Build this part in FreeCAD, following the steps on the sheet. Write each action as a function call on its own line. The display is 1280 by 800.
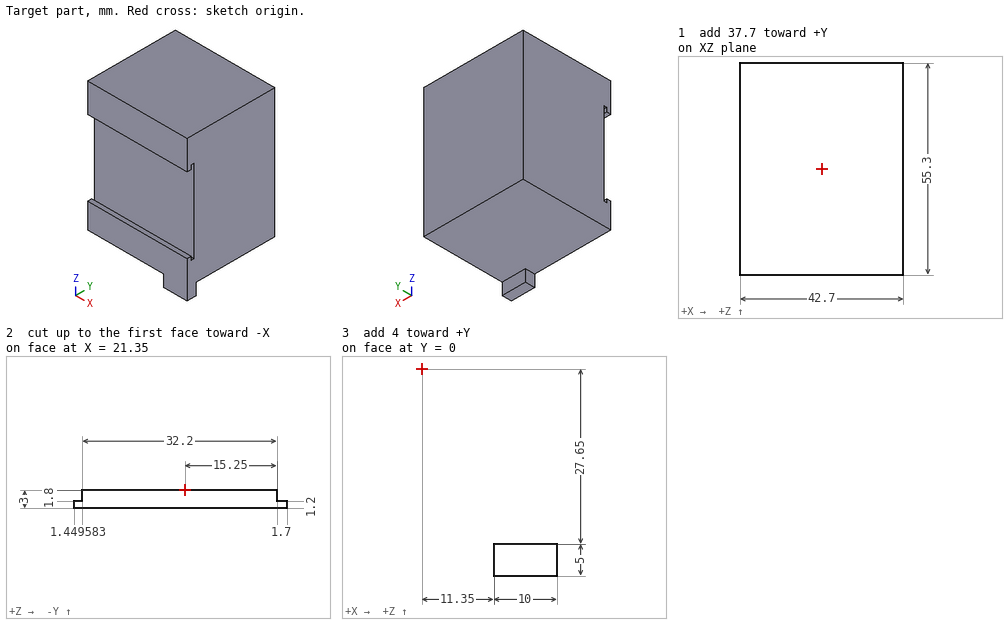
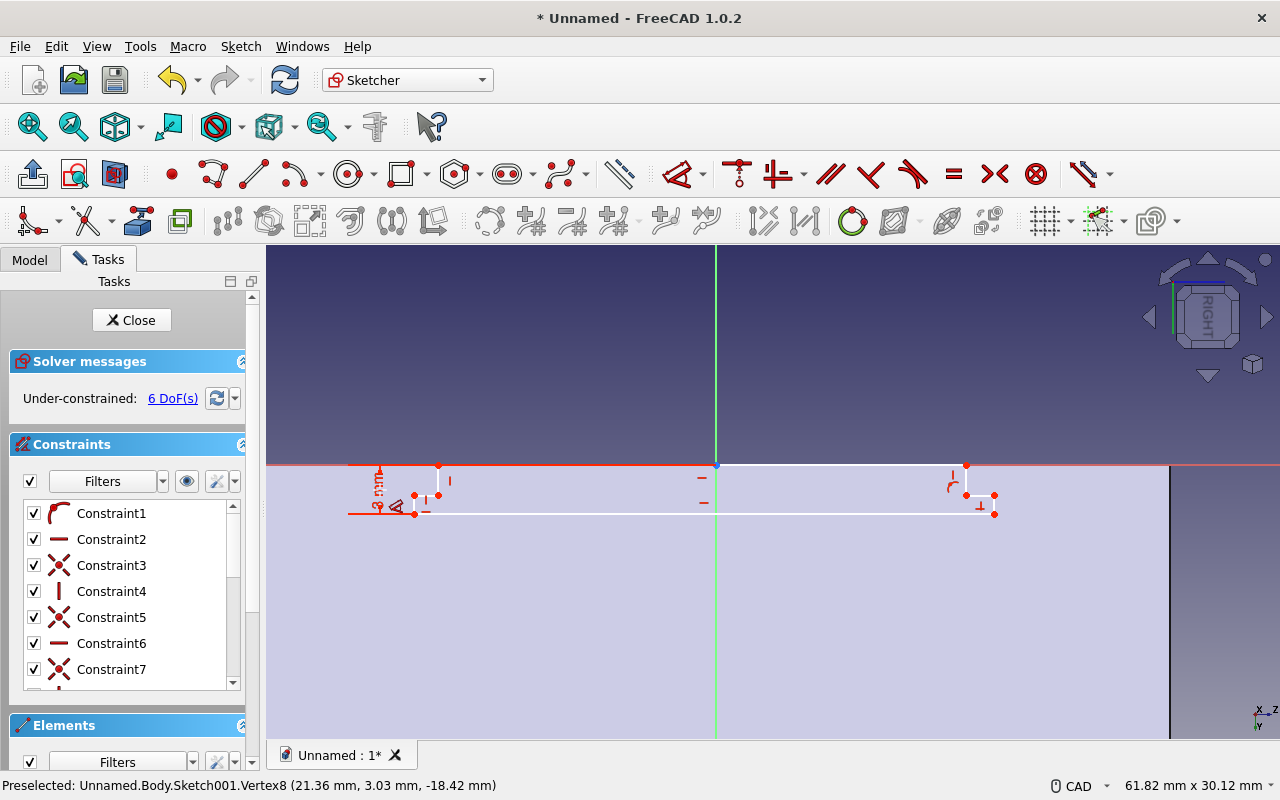
scroll(438, 474, up, 3)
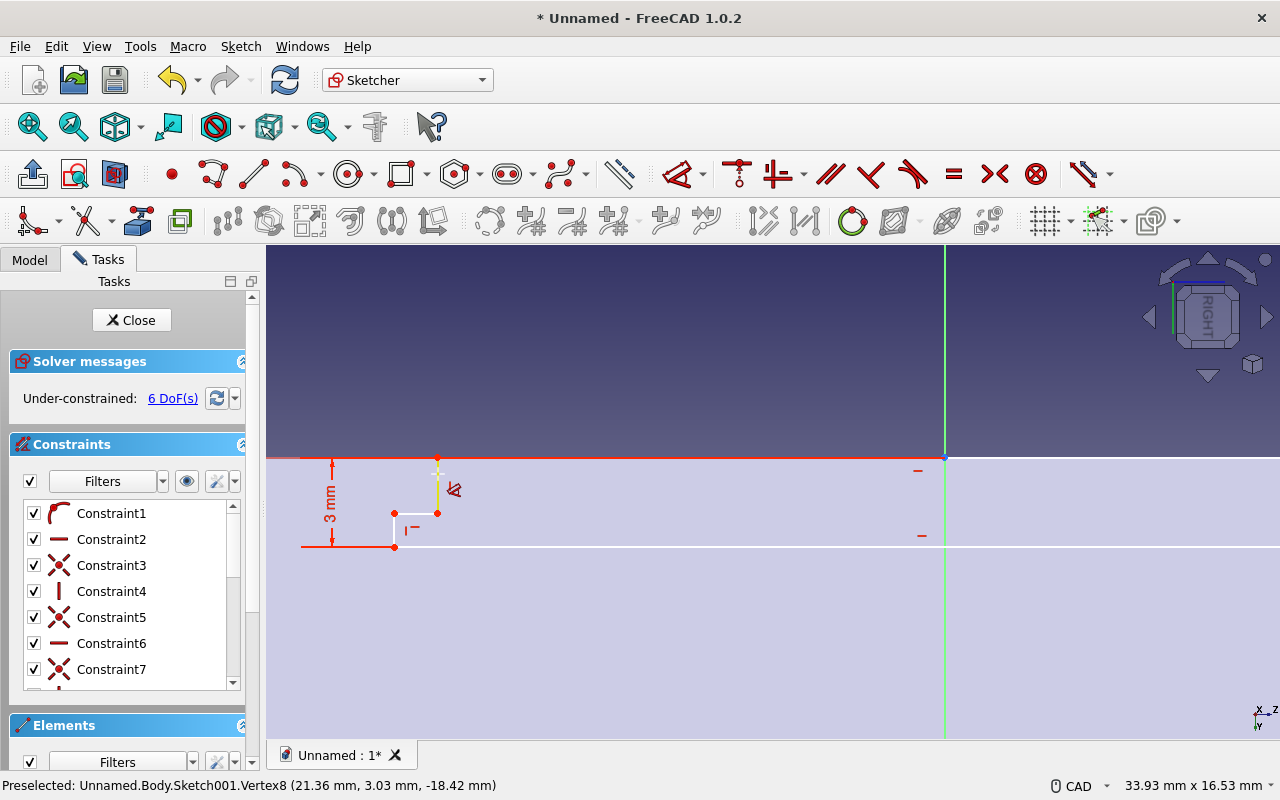
click(438, 475)
click(404, 486)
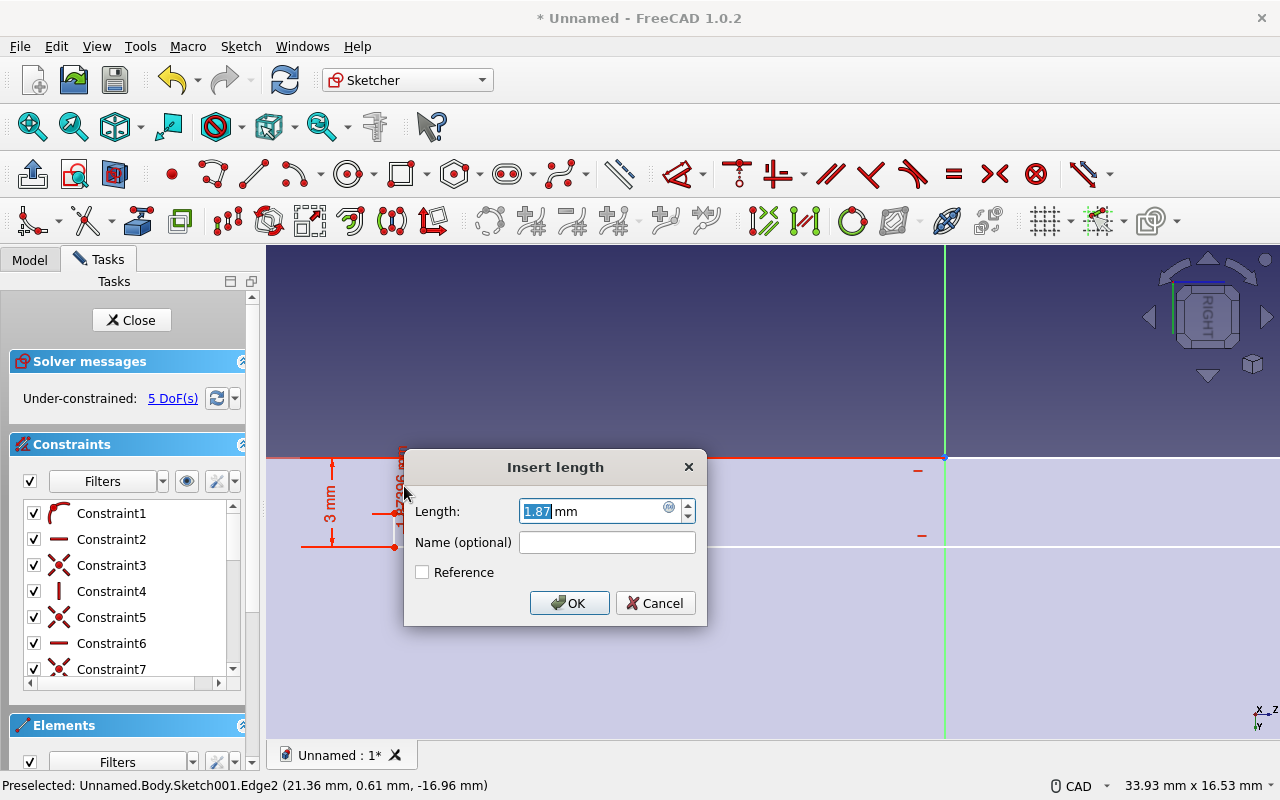
text(1.8)
key(Return)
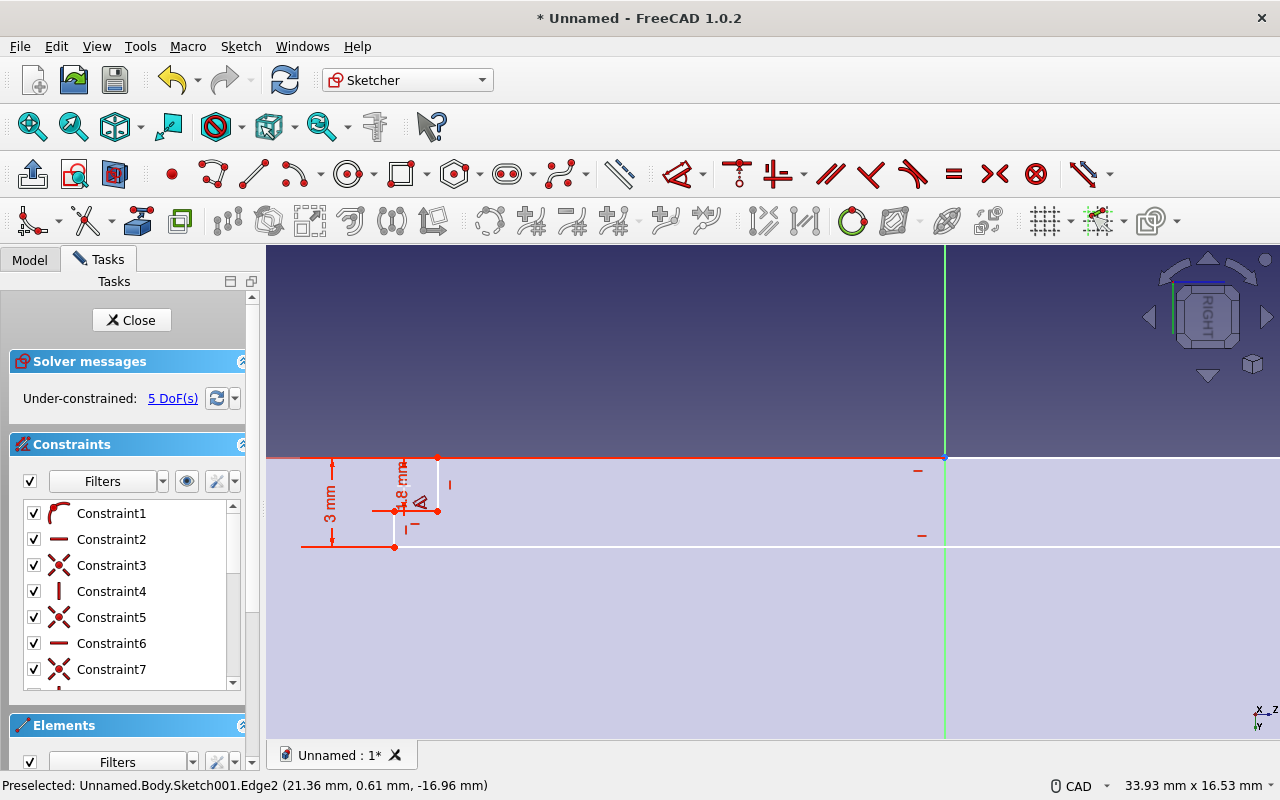
scroll(439, 479, down, 3)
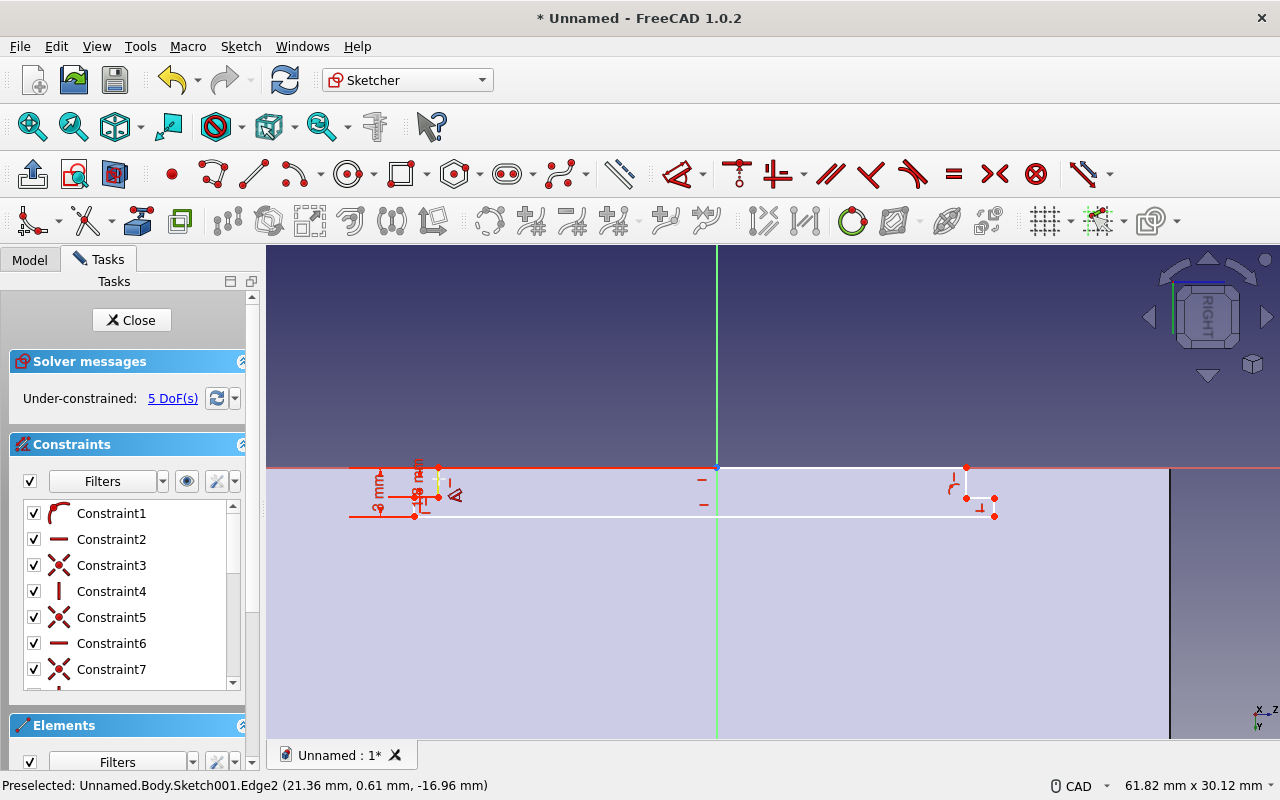
scroll(994, 511, up, 5)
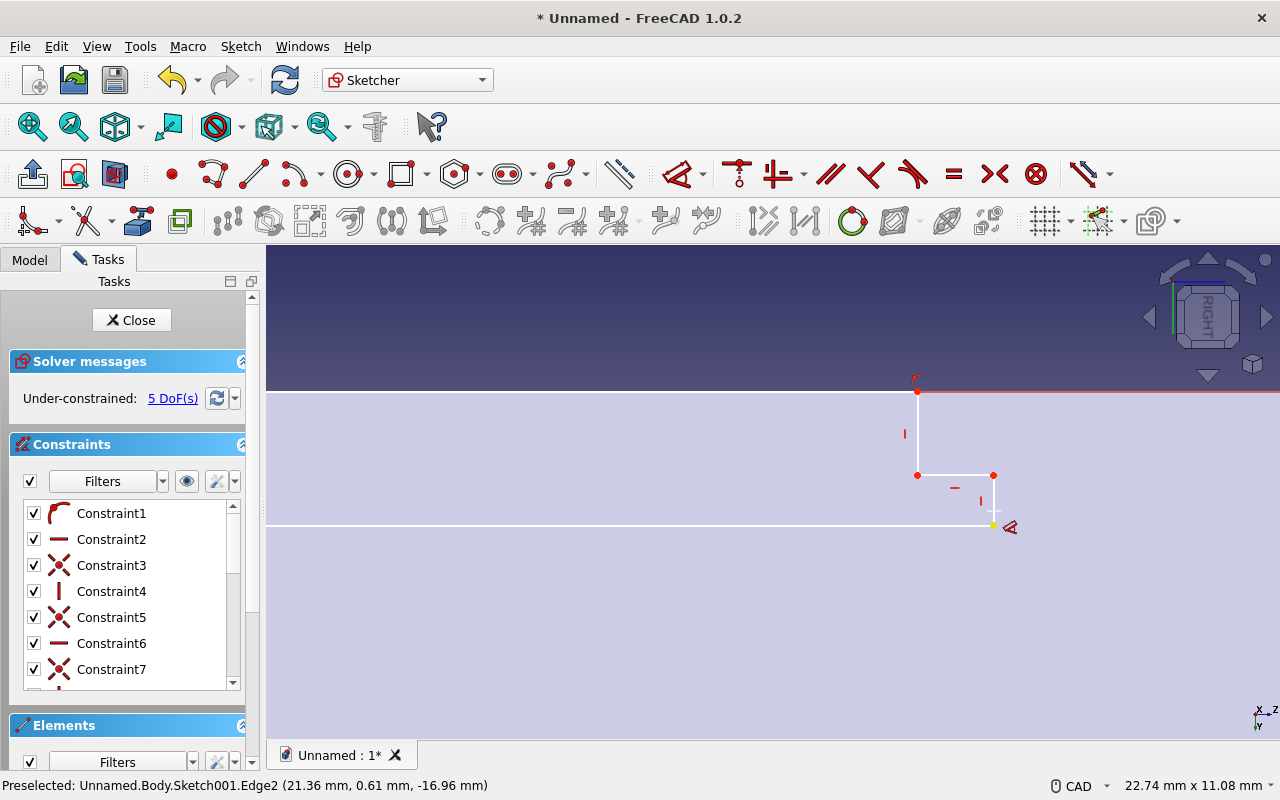
click(994, 511)
click(1028, 501)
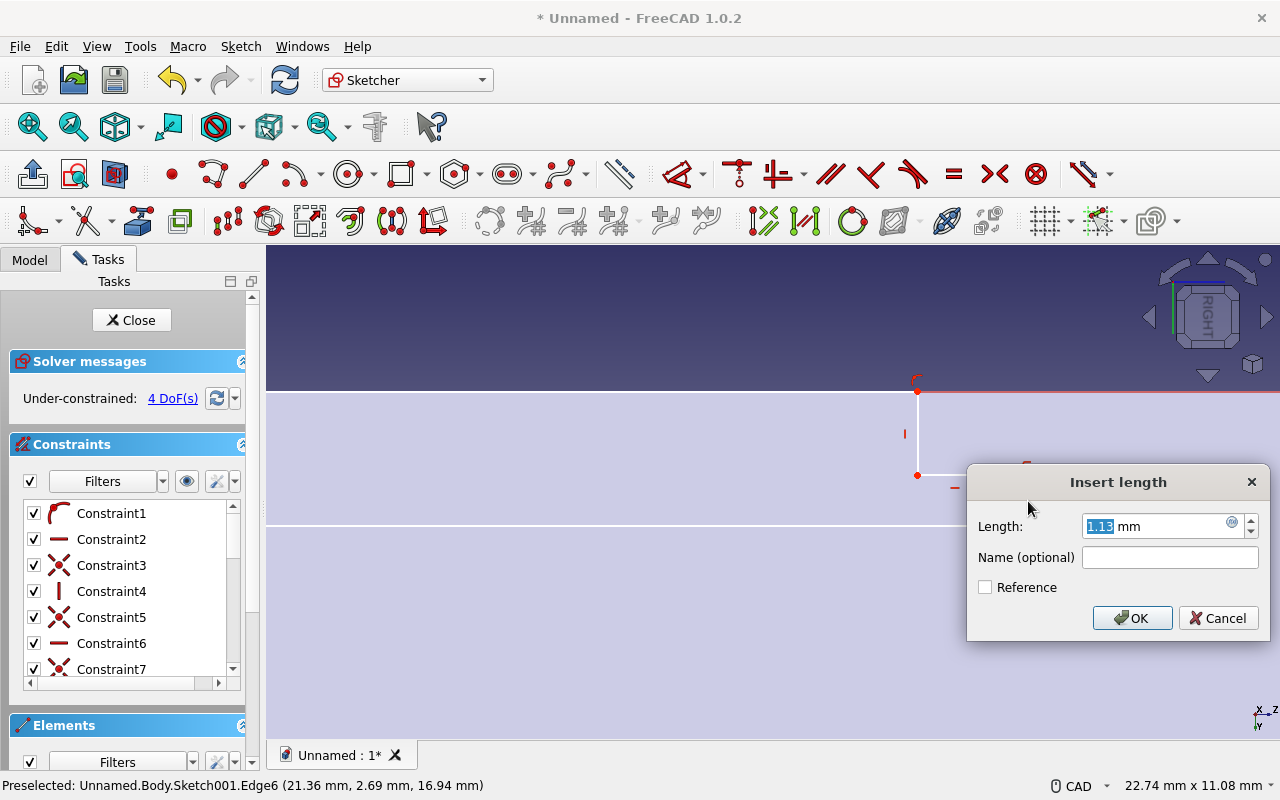
text(1.2)
key(Return)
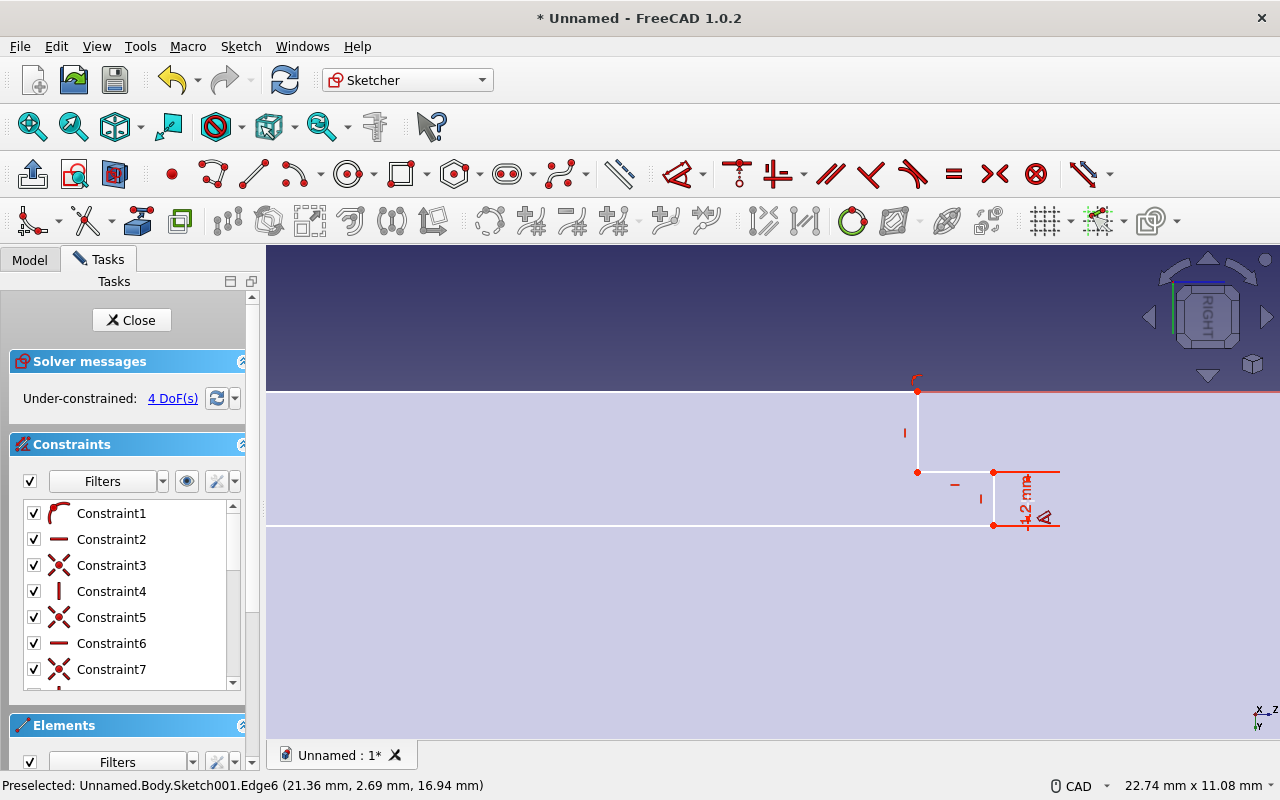
click(971, 472)
click(956, 506)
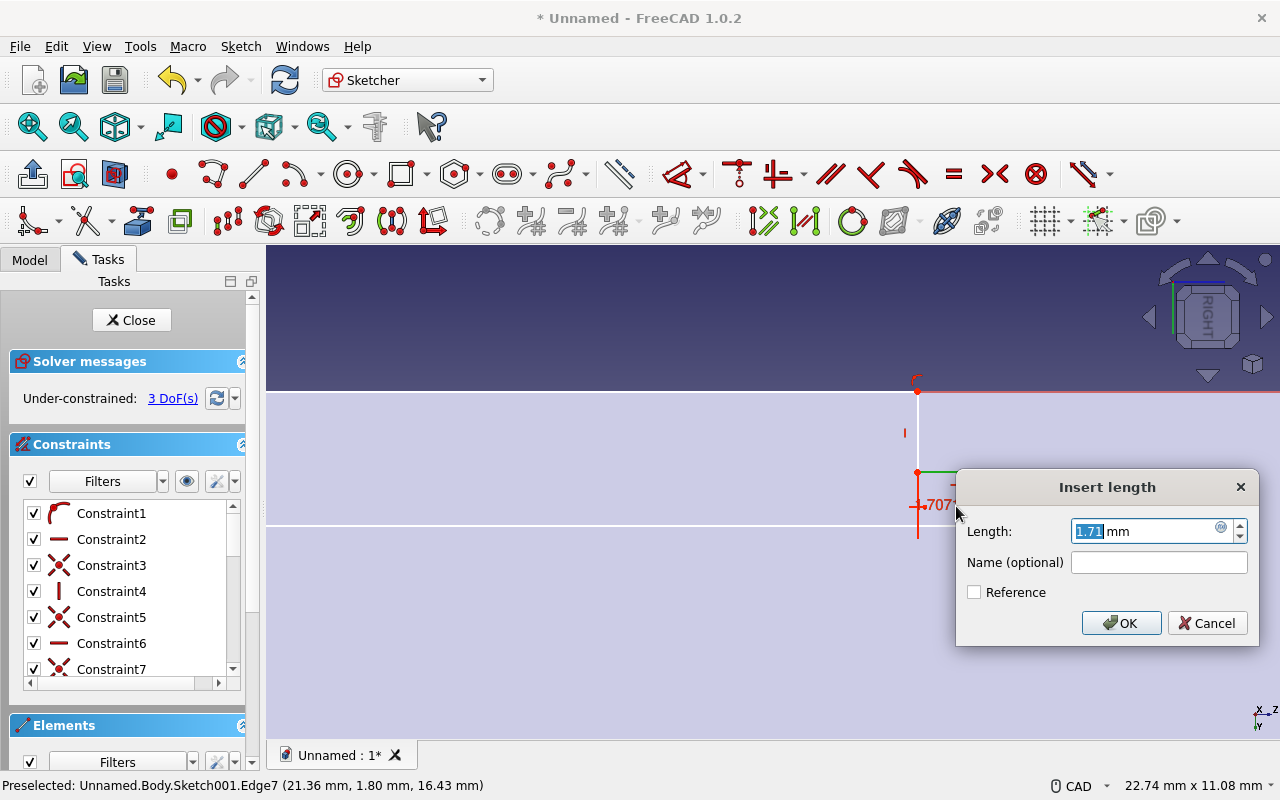
text(1.7)
key(Return)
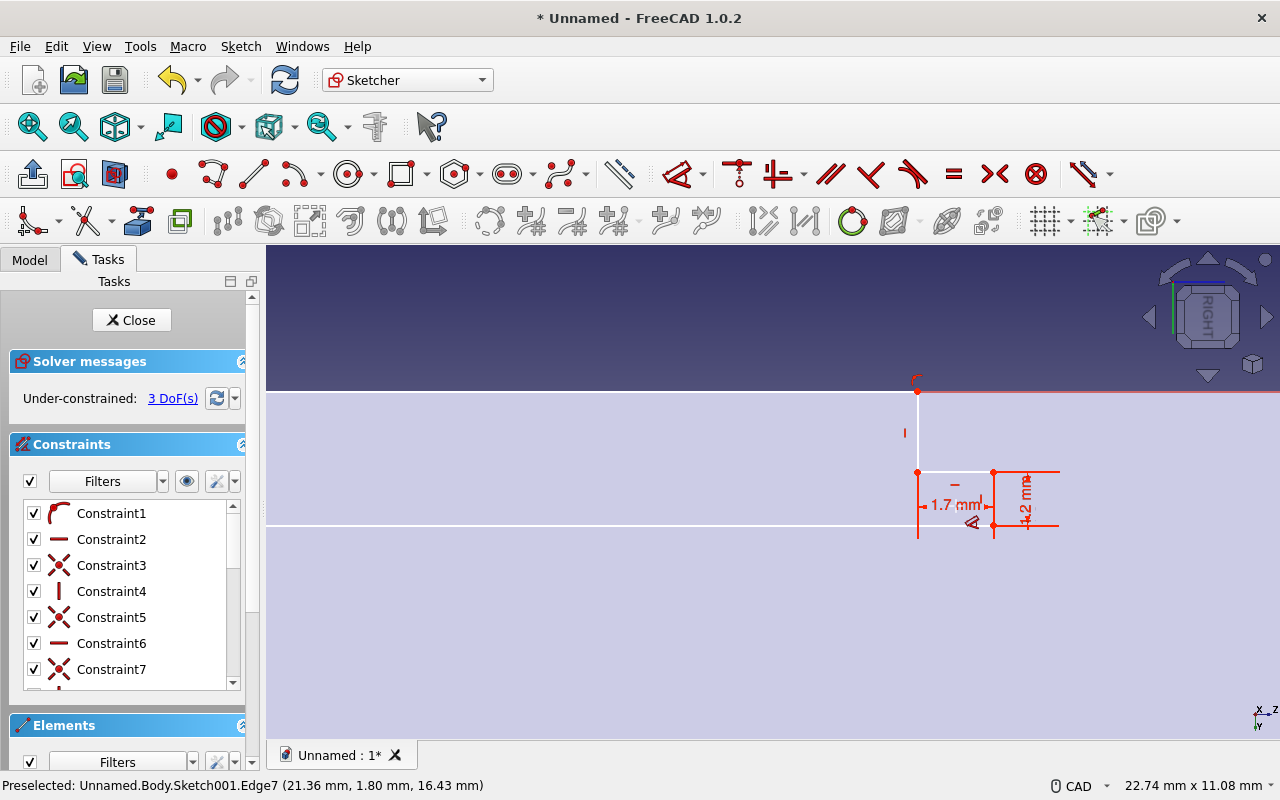
click(487, 392)
click(606, 358)